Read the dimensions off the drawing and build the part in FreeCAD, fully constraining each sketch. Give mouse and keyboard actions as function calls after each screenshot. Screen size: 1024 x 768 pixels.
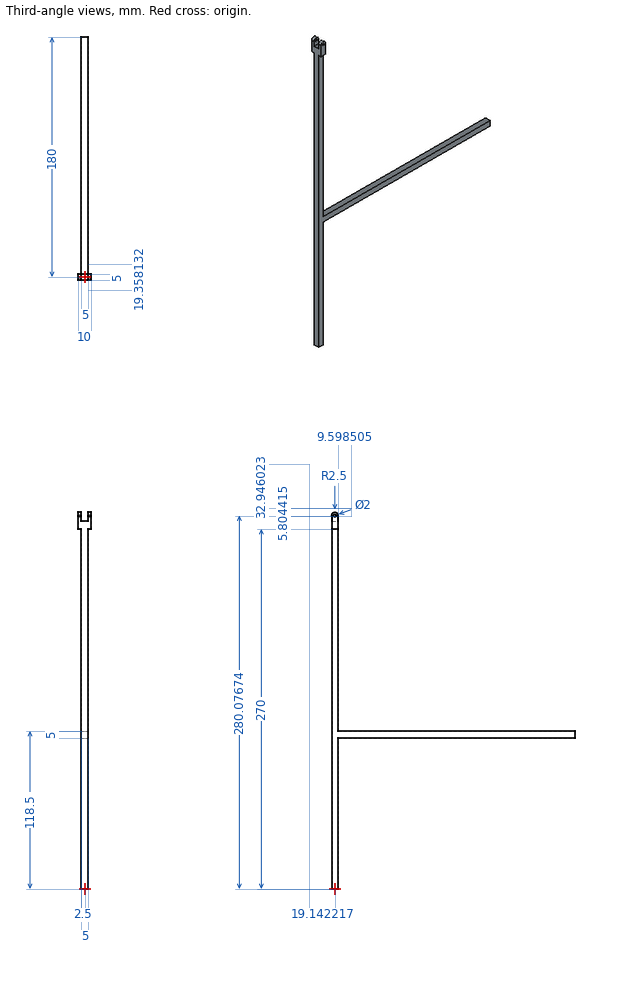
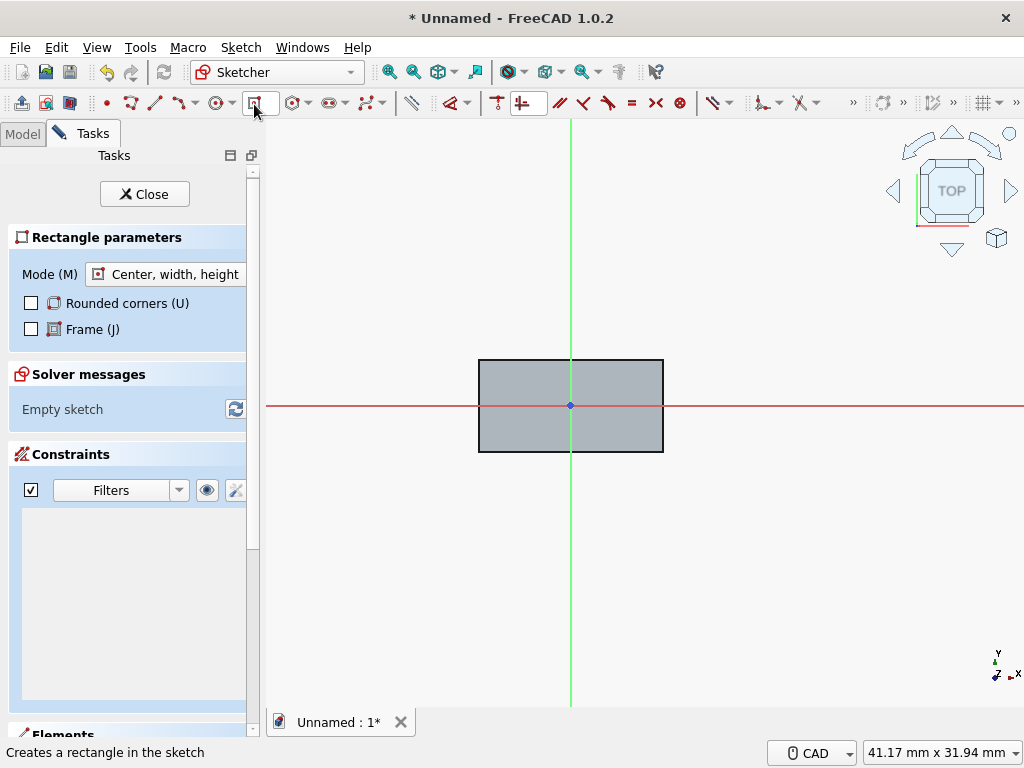
click(571, 406)
click(617, 227)
key(Escape)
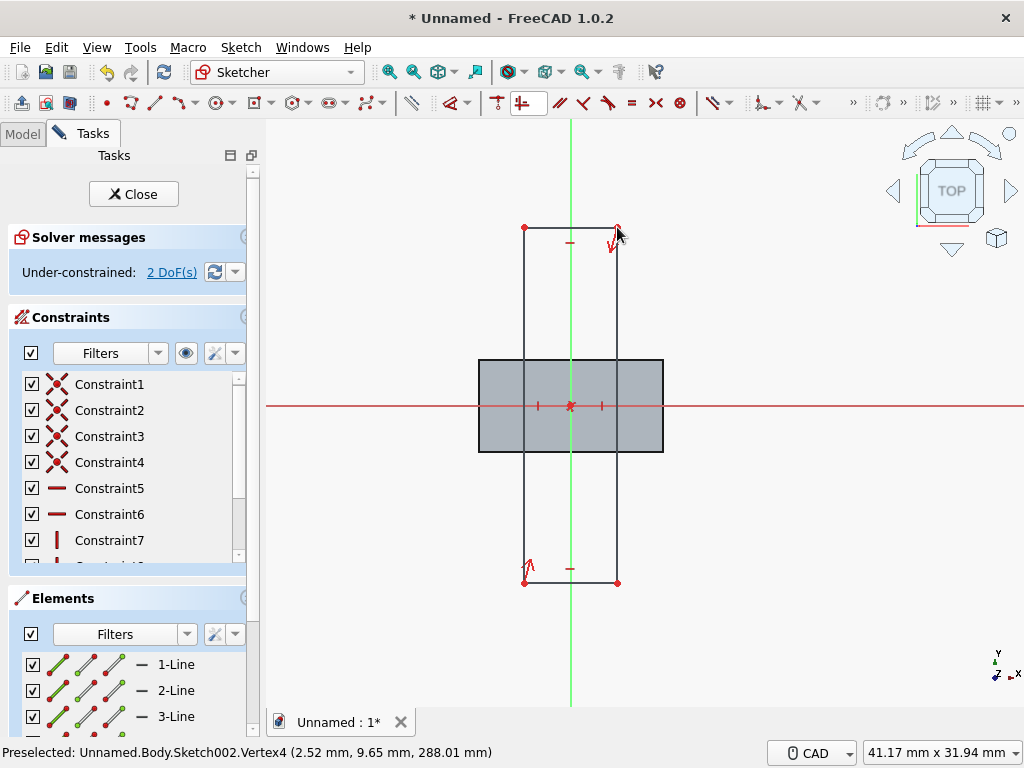
click(450, 104)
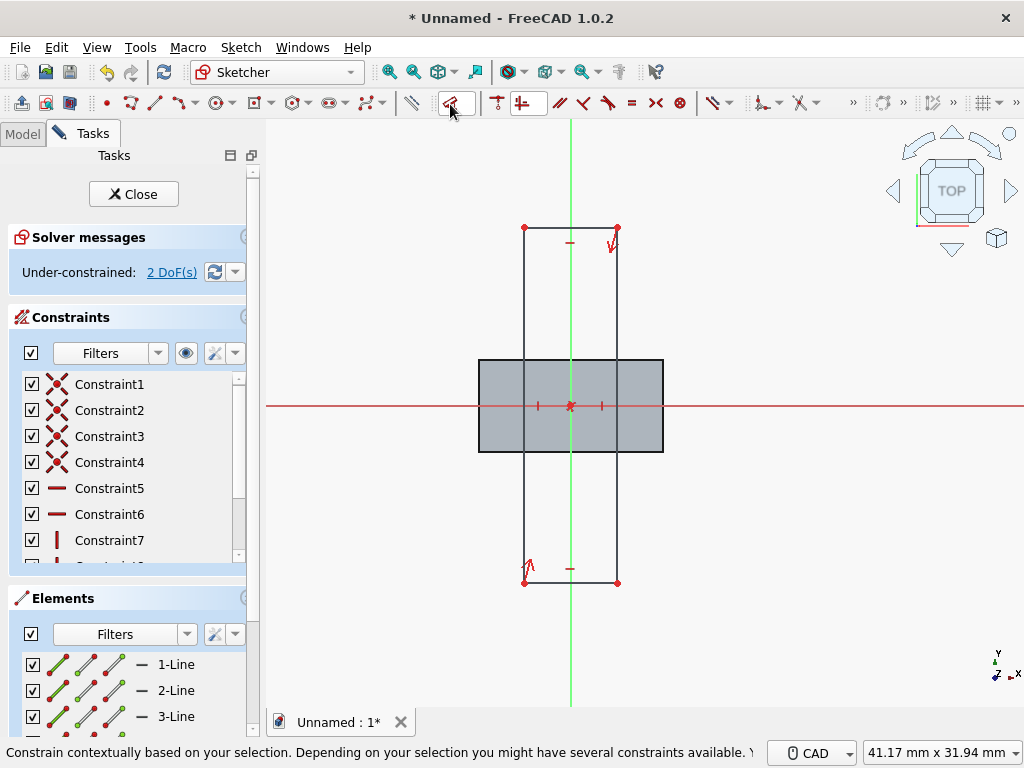
click(552, 583)
click(549, 617)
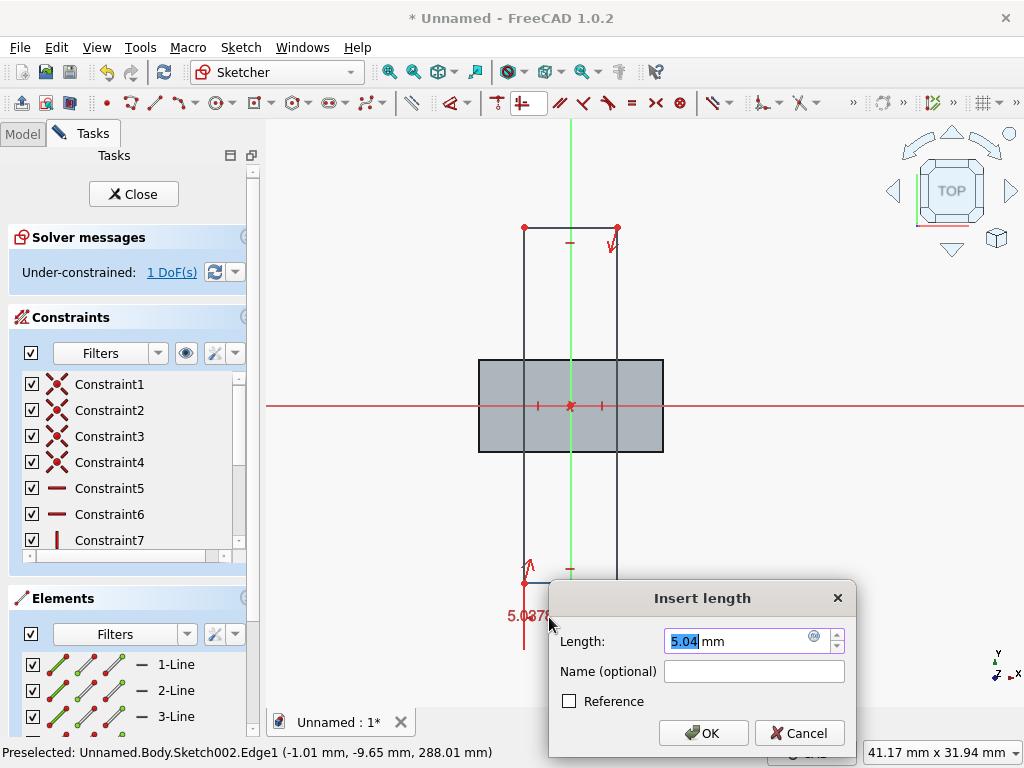
text(5)
key(Return)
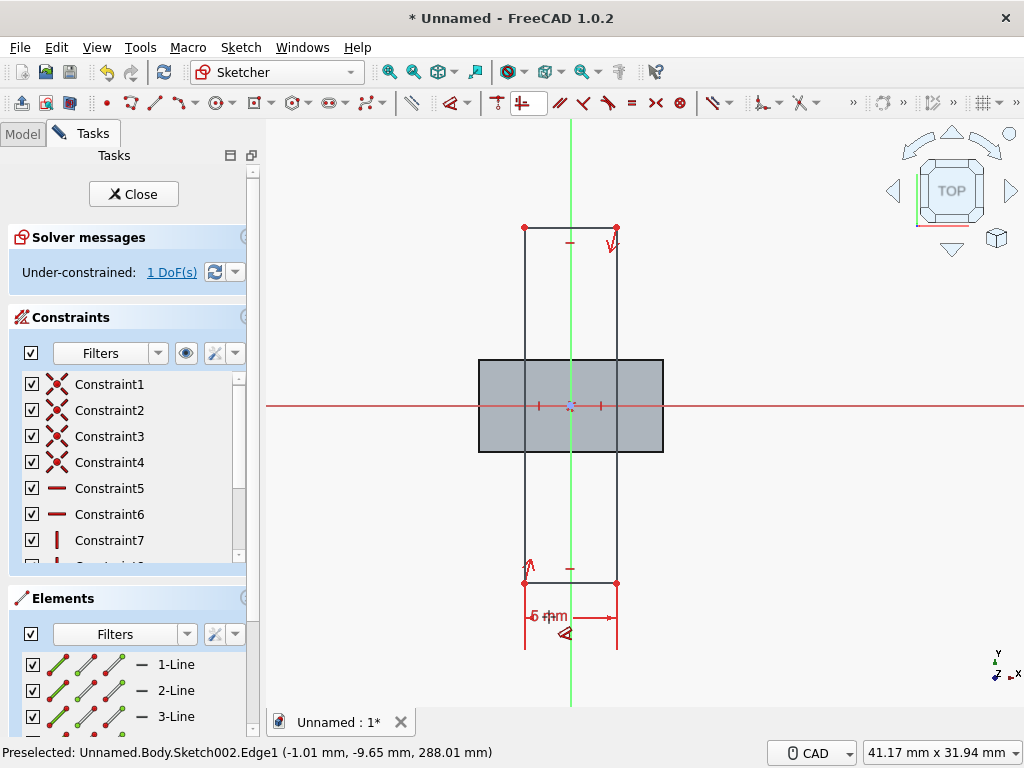
click(617, 477)
click(651, 324)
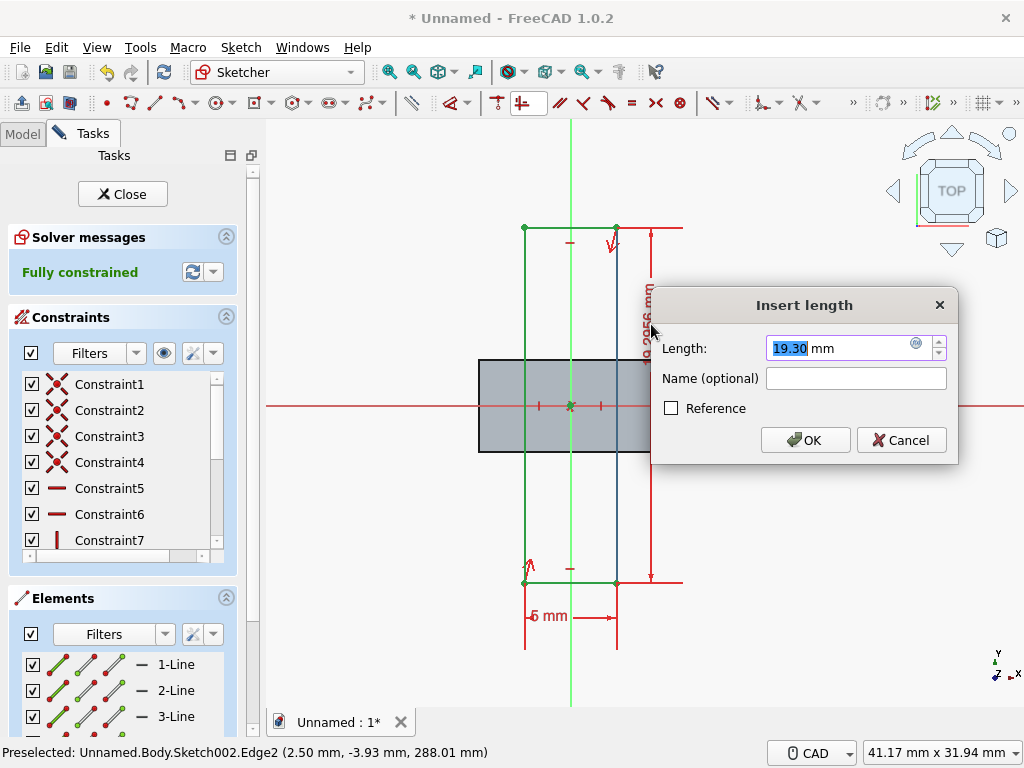
text(19.358132)
key(Return)
key(Escape)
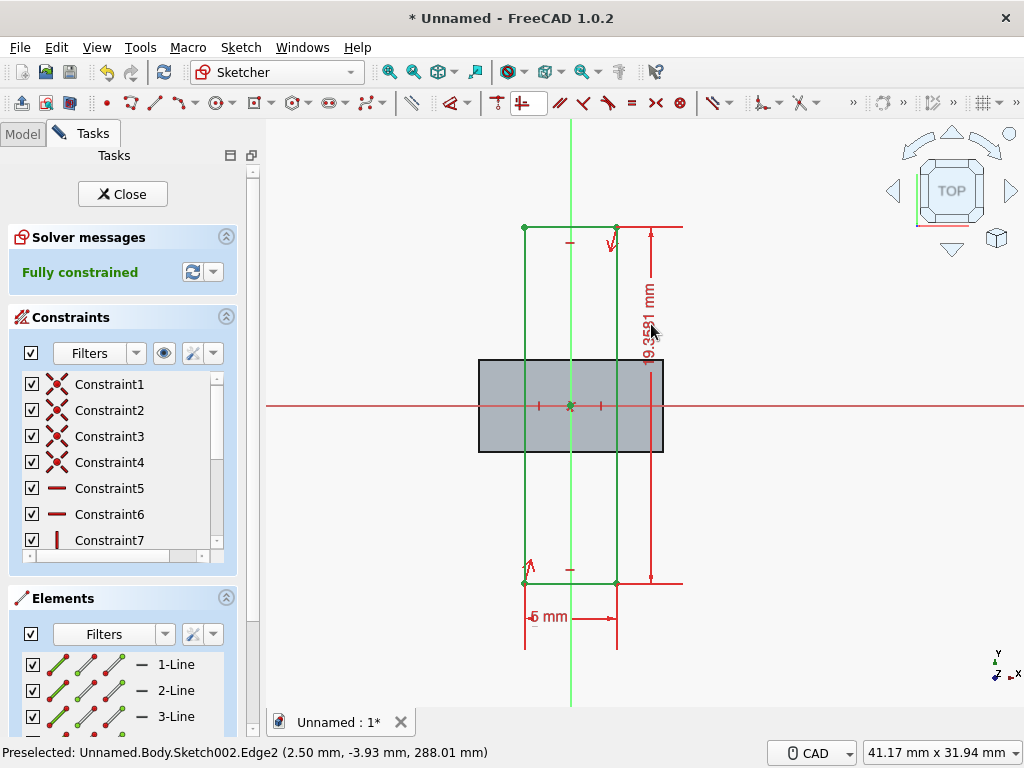
click(123, 194)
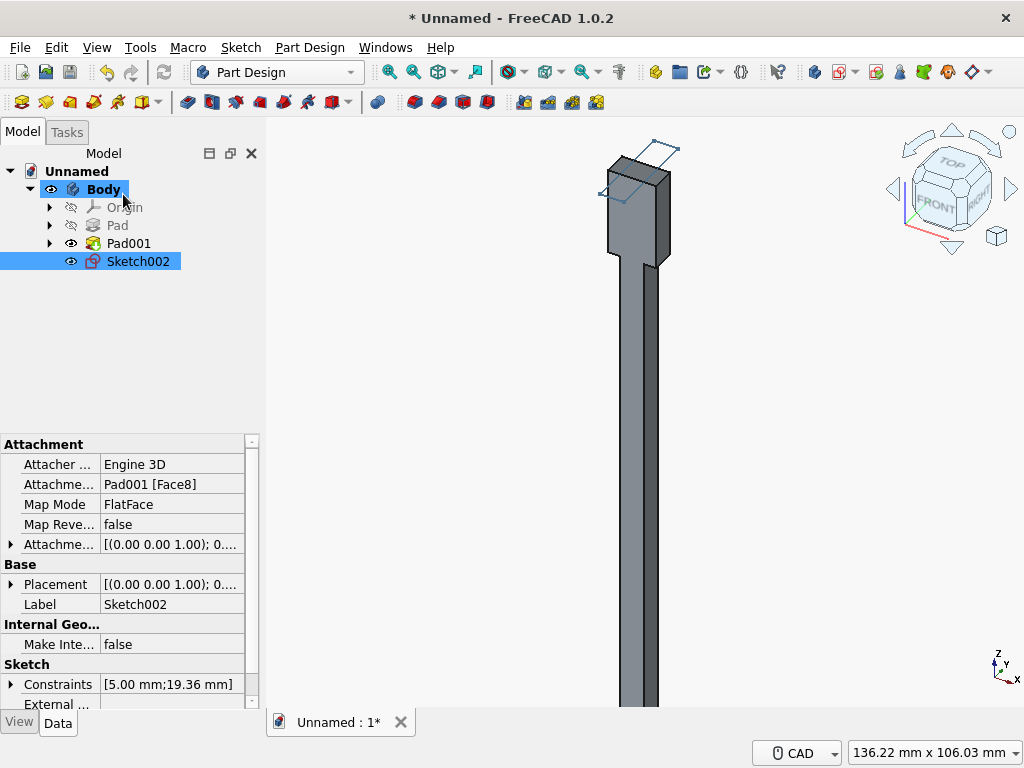
click(188, 102)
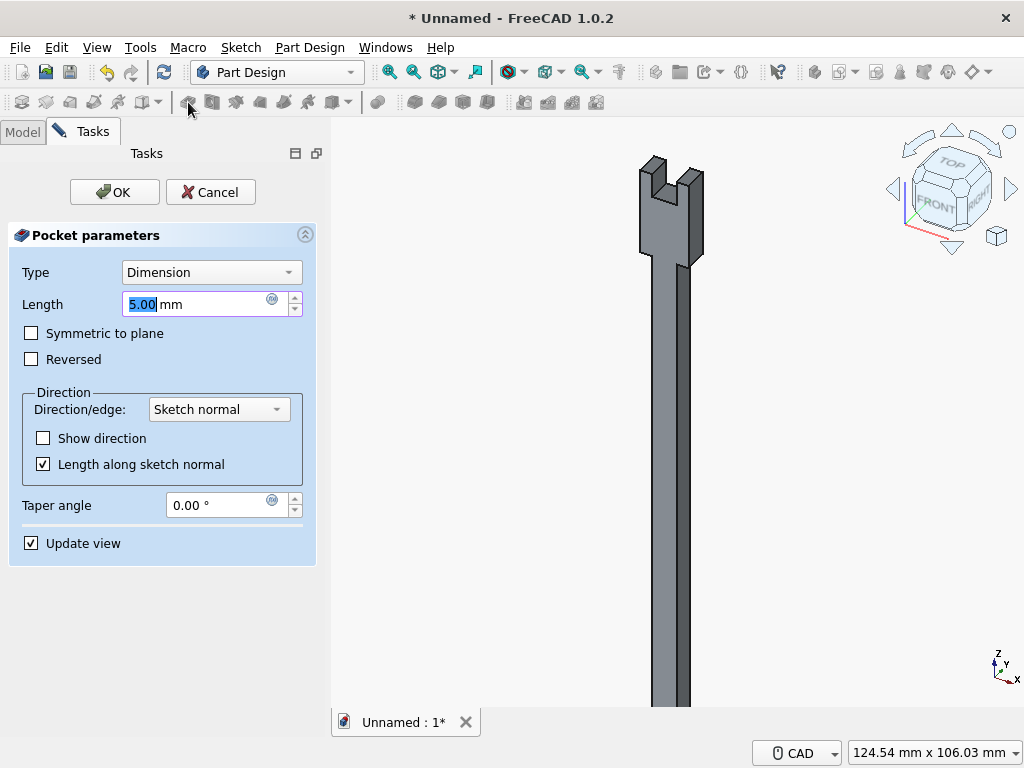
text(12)
key(Tab)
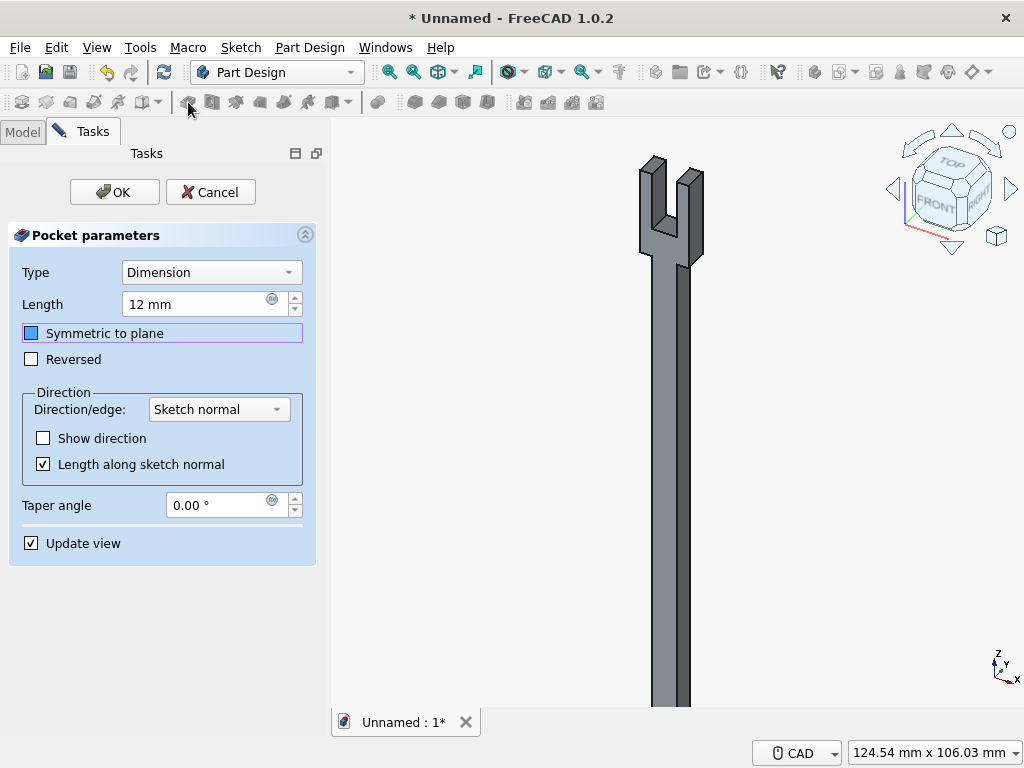
click(115, 192)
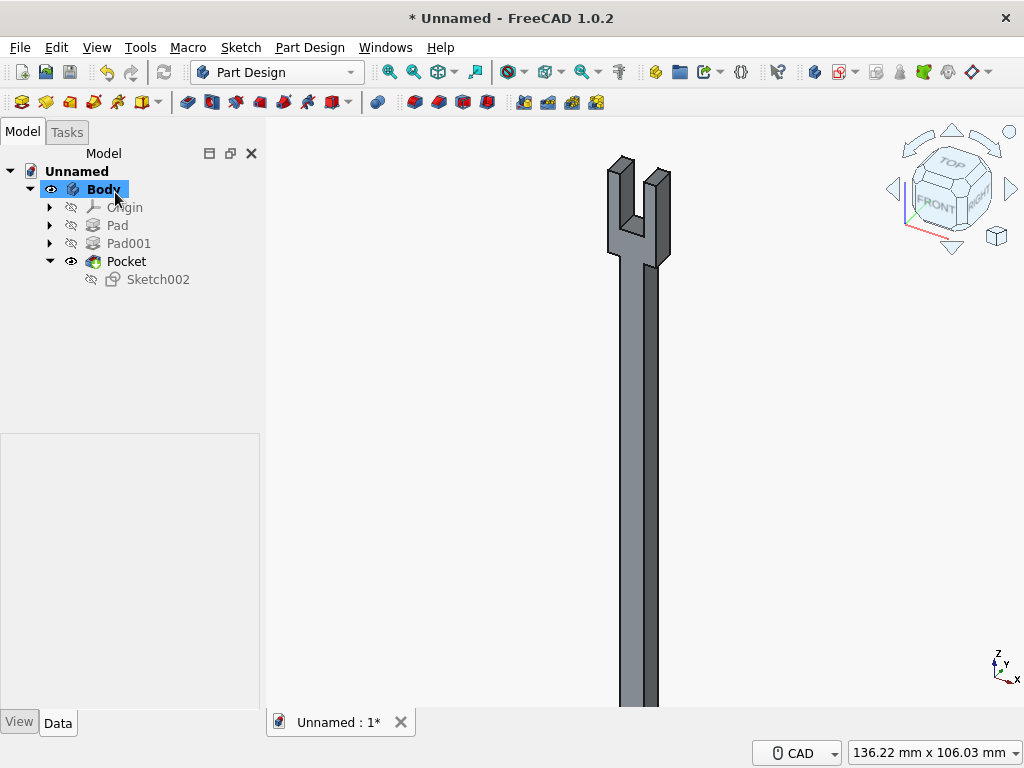
click(390, 72)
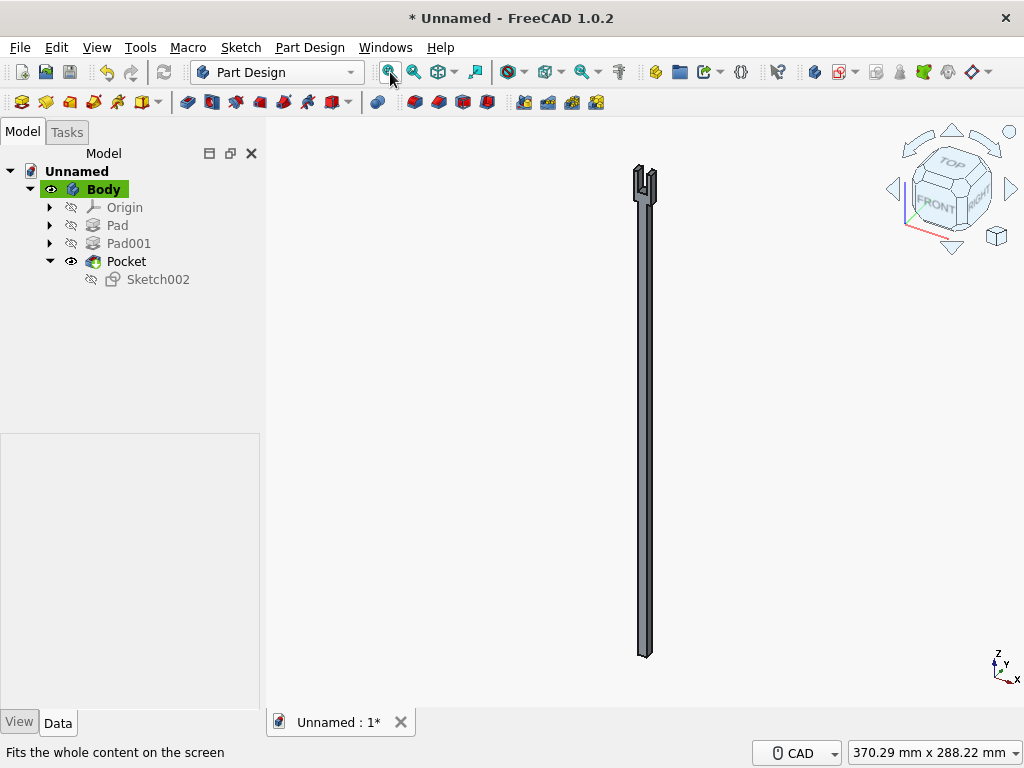
scroll(654, 179, up, 5)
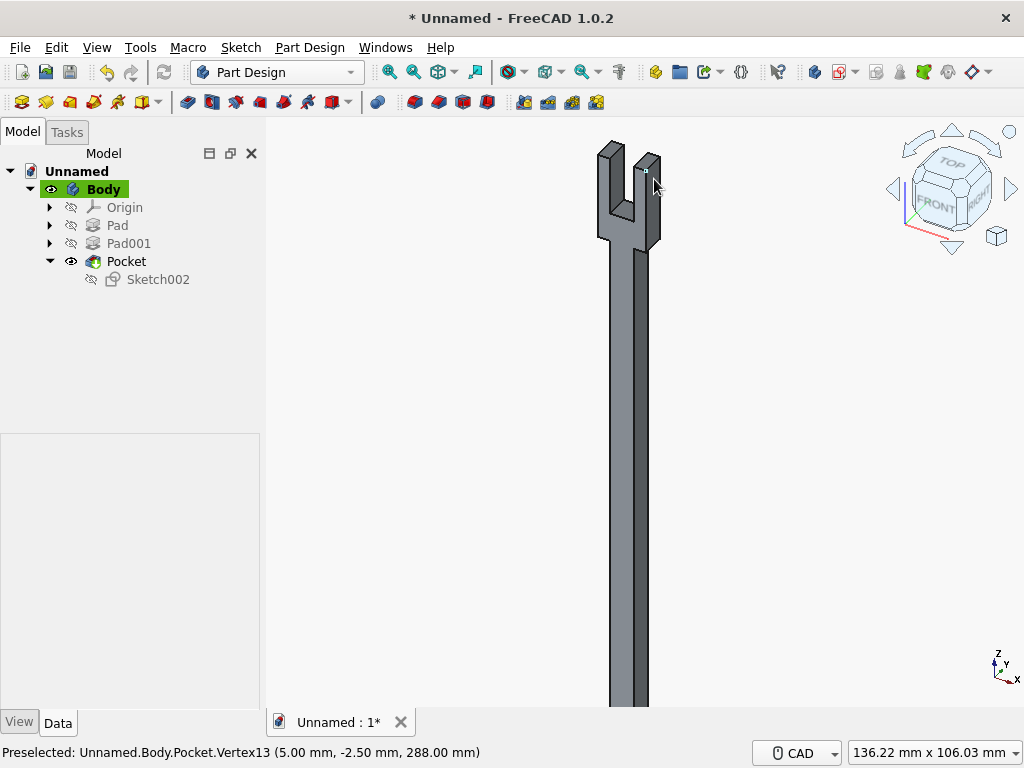
click(390, 72)